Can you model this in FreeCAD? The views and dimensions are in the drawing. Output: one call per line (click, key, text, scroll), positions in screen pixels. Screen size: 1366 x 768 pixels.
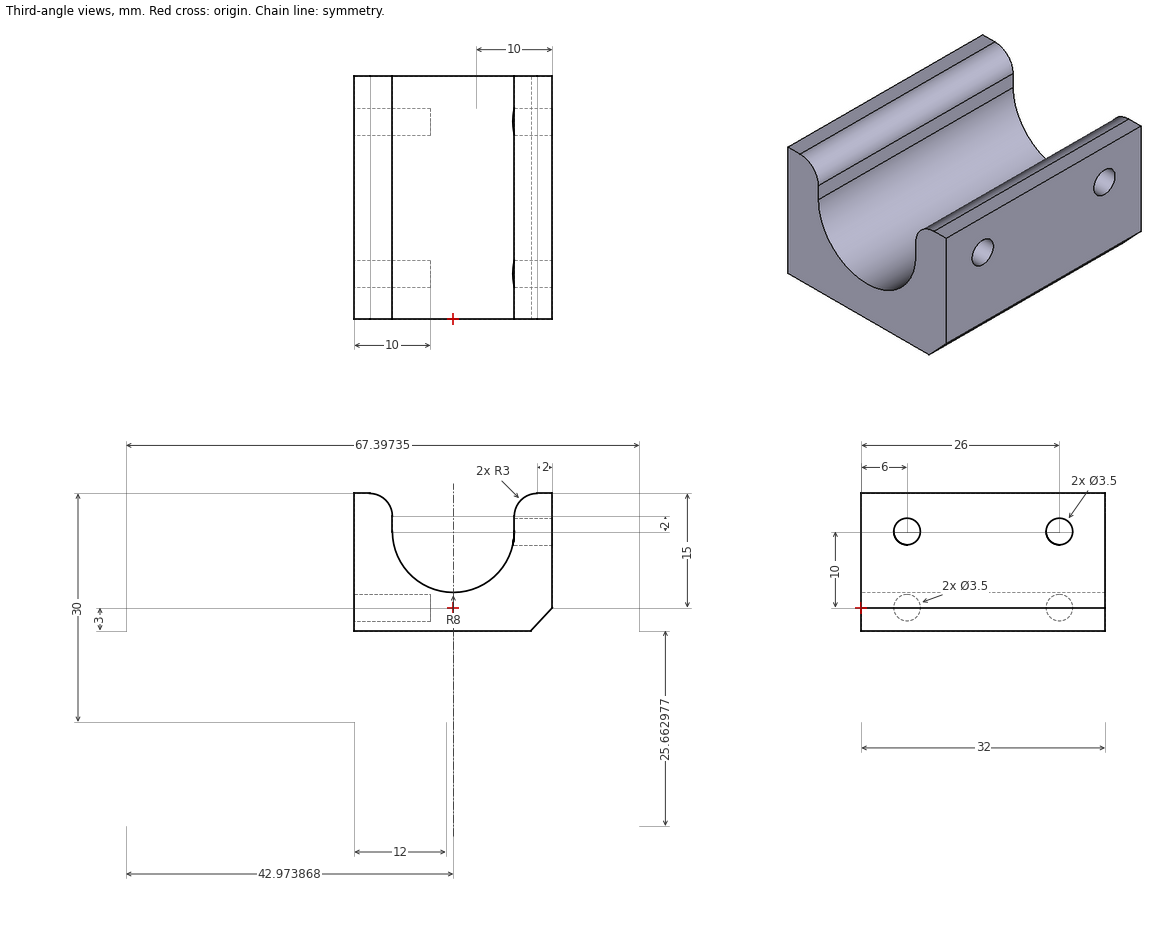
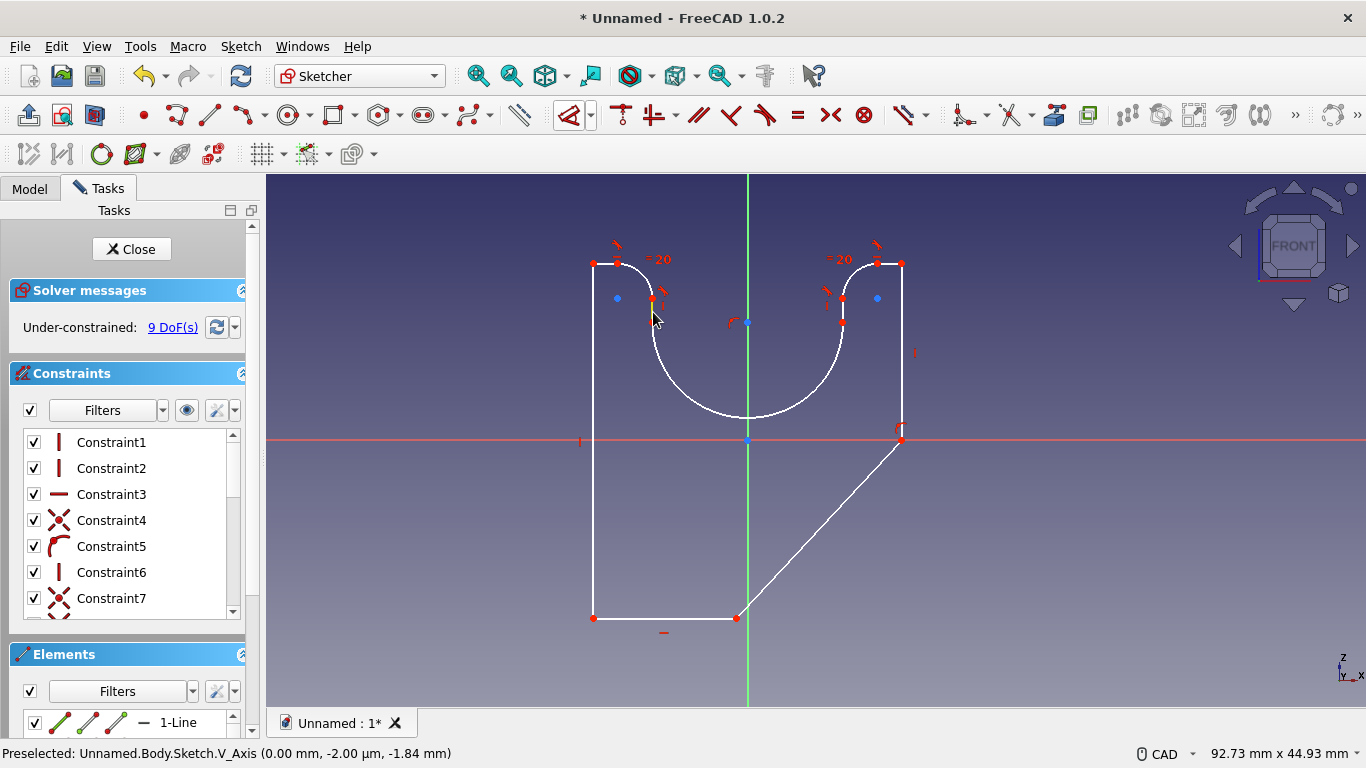
click(902, 264)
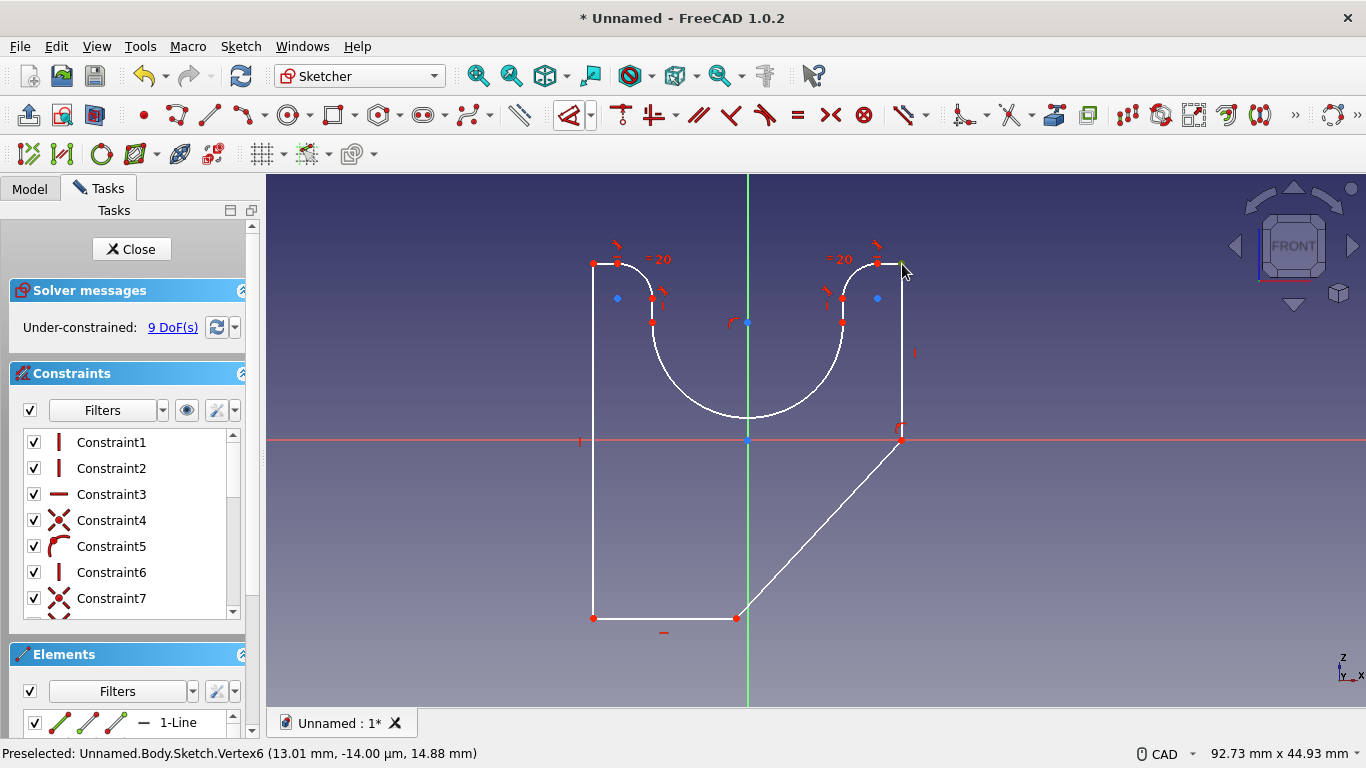
click(593, 264)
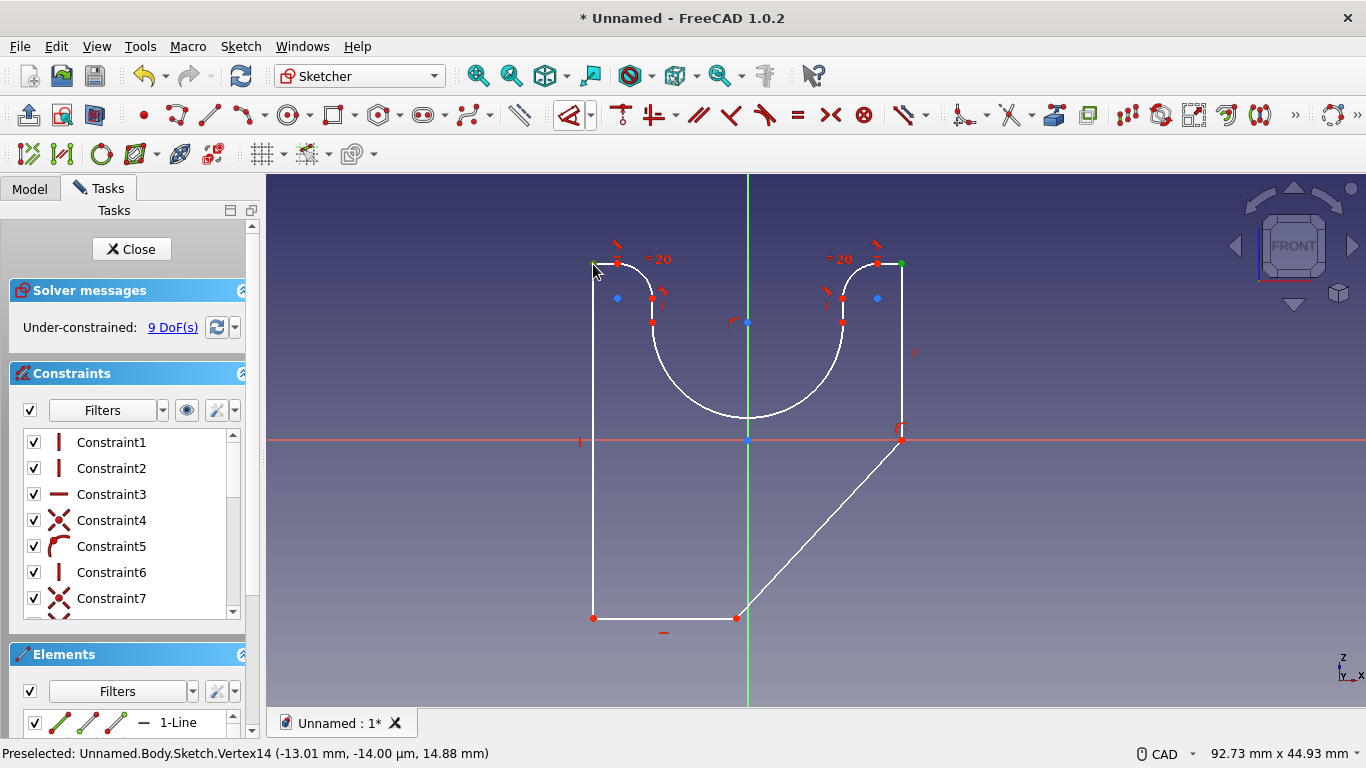
click(748, 543)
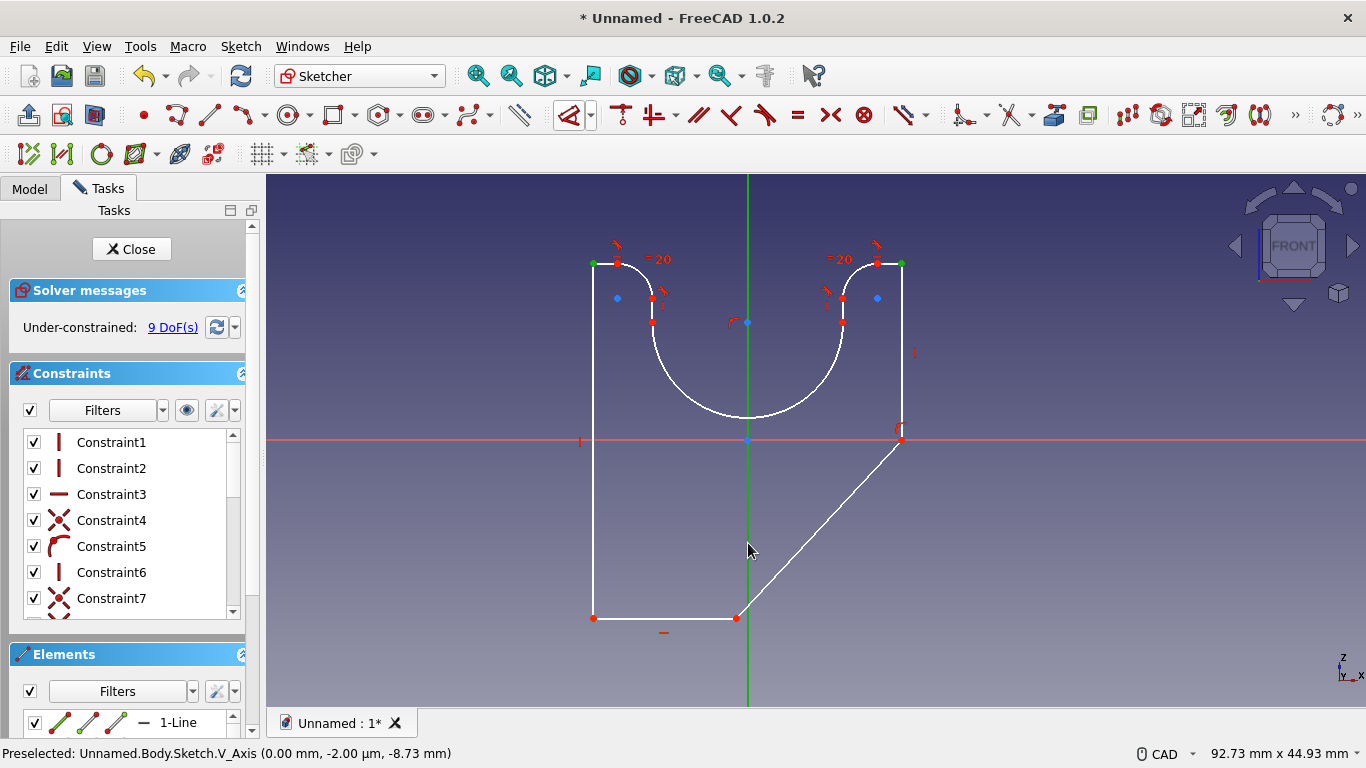
click(831, 116)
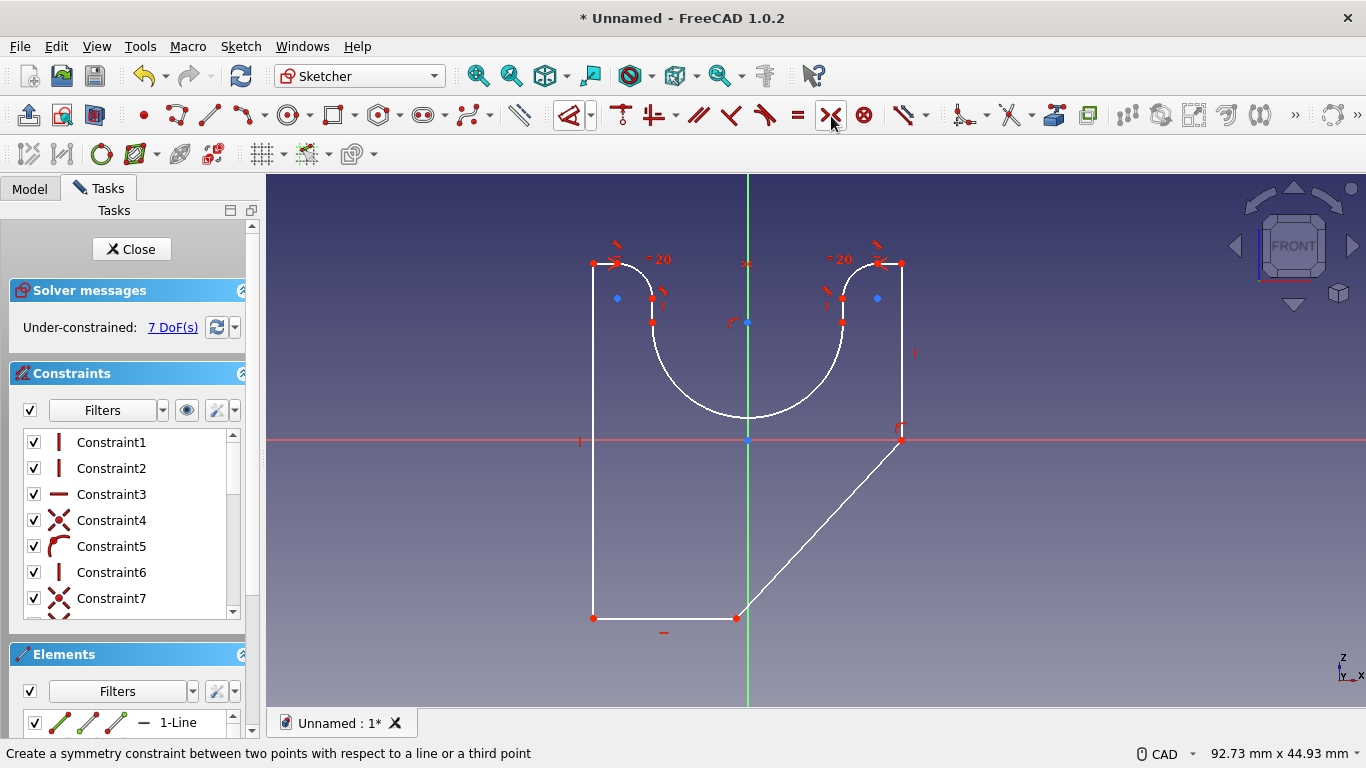
click(568, 116)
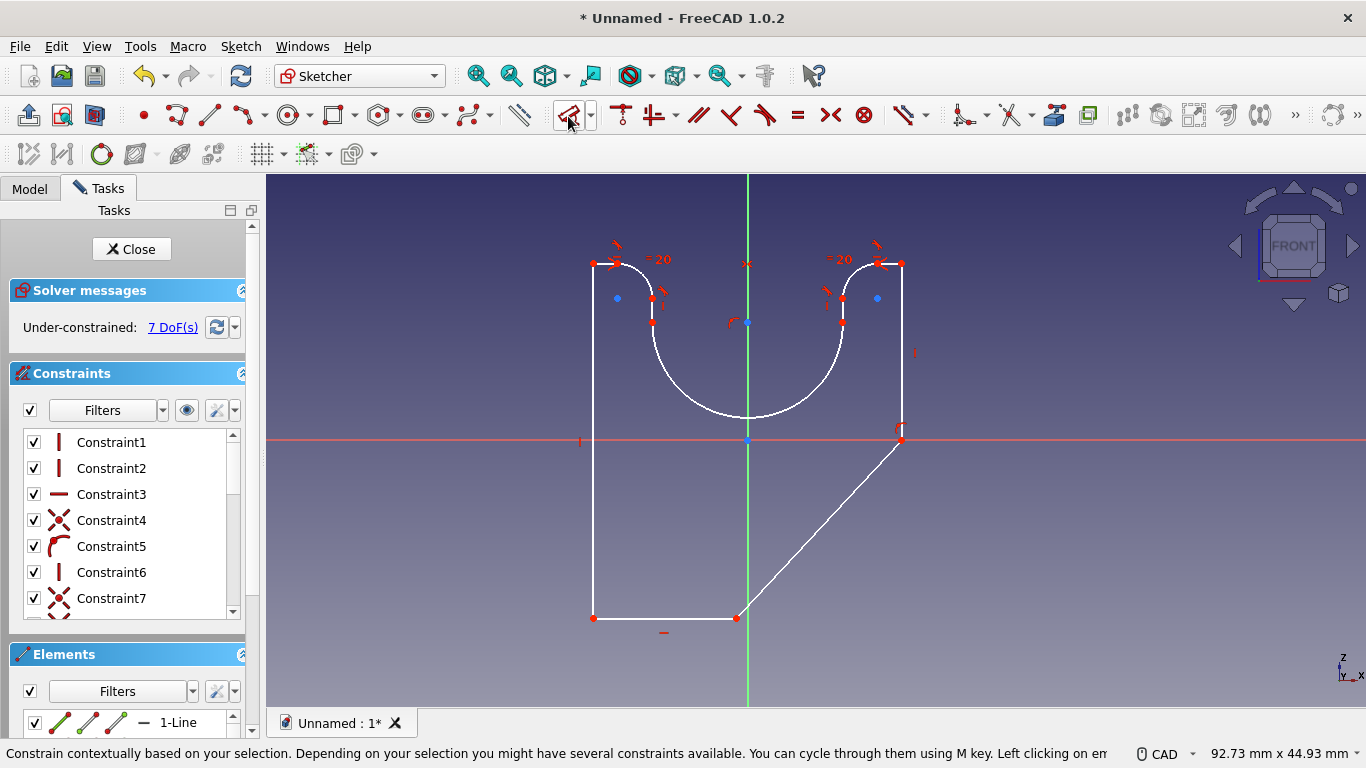
click(692, 400)
click(673, 426)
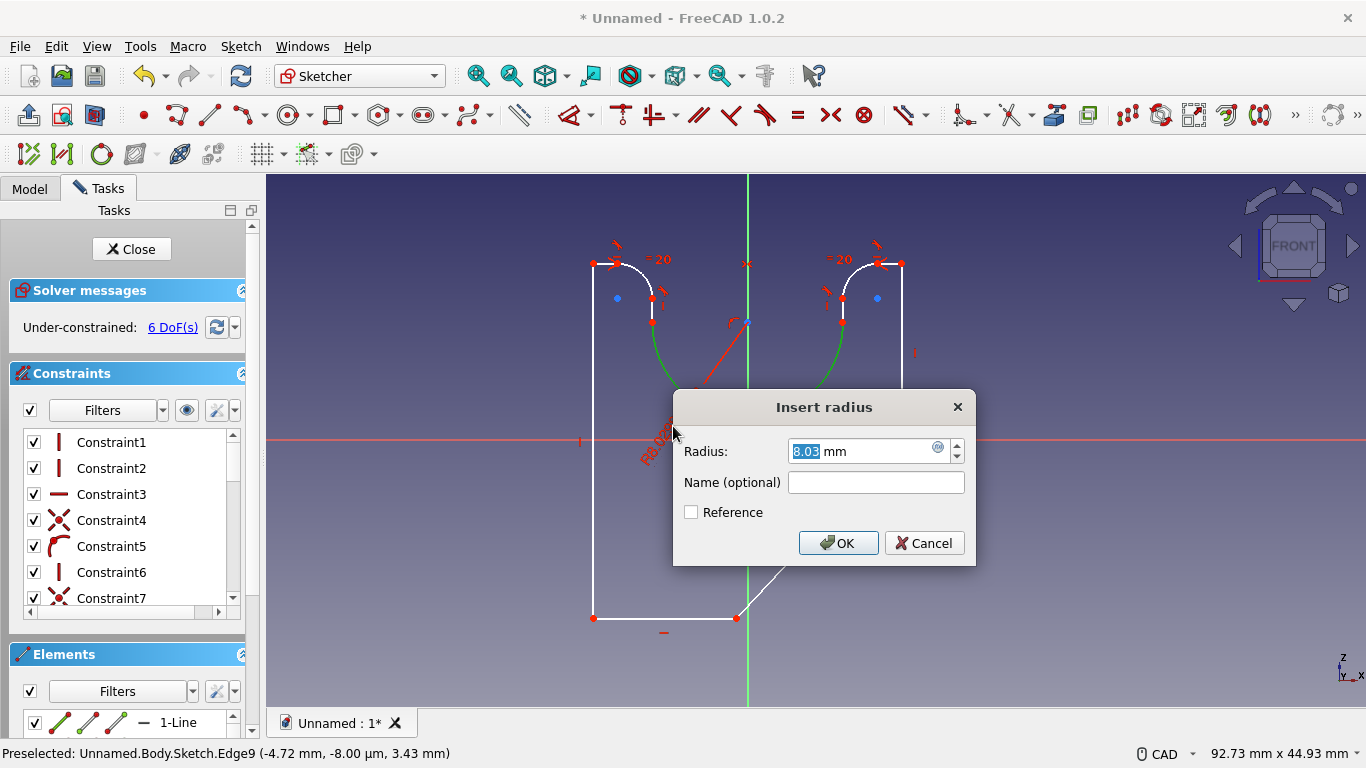
text(8)
key(Return)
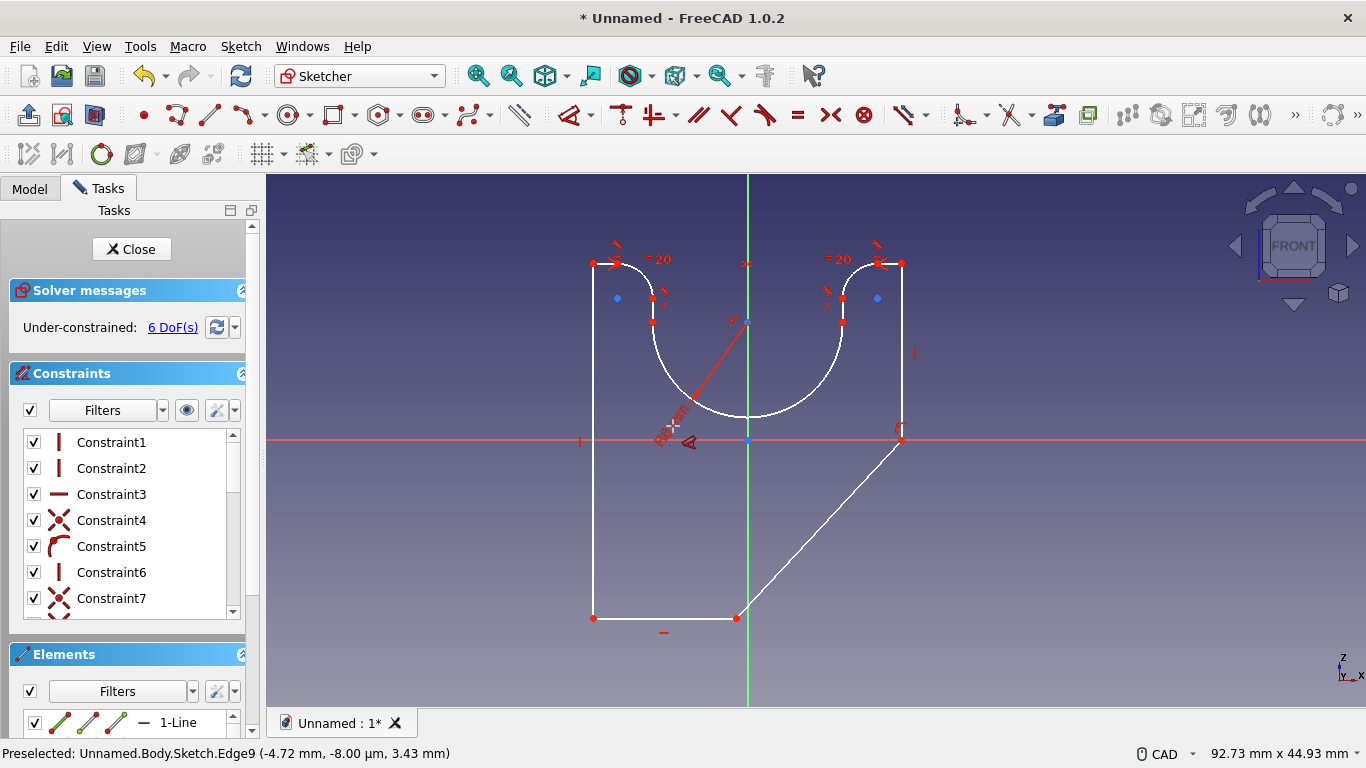
click(862, 268)
click(848, 239)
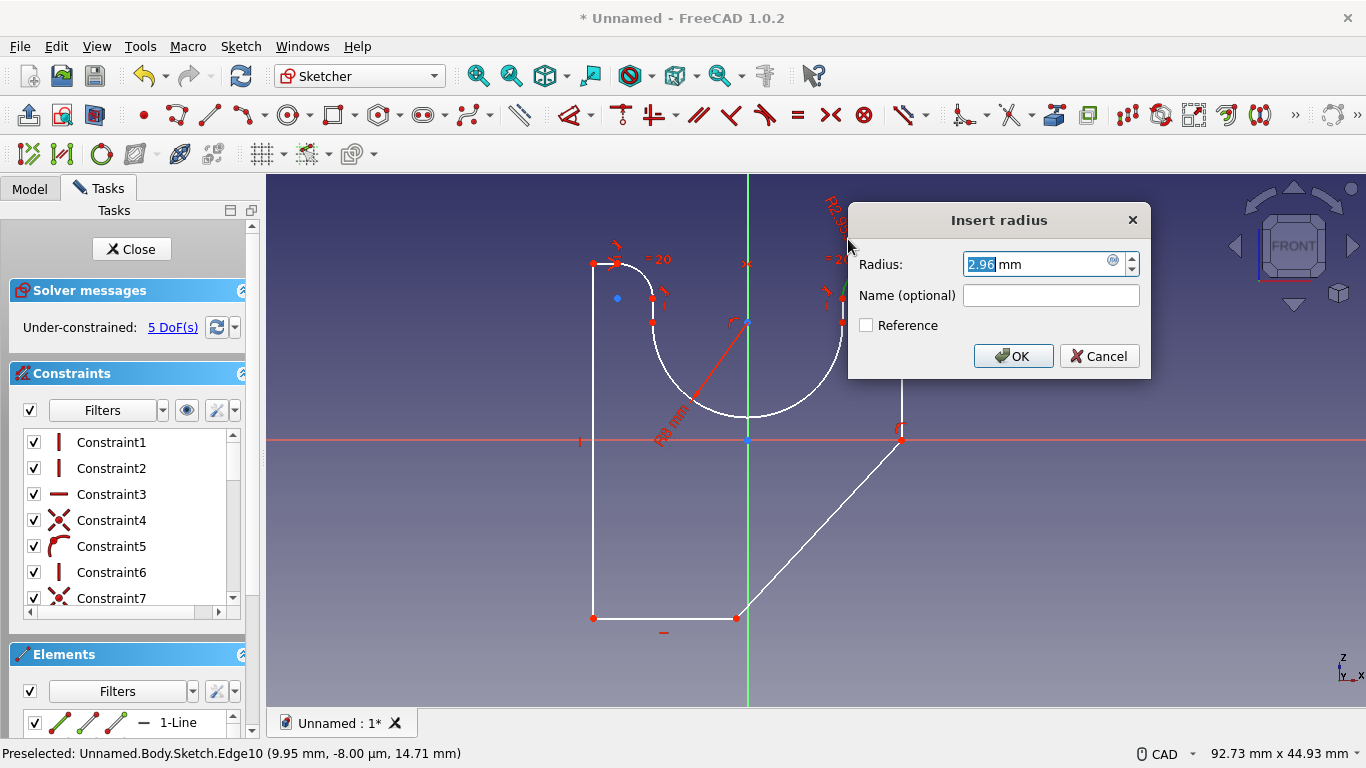
text(3)
key(Return)